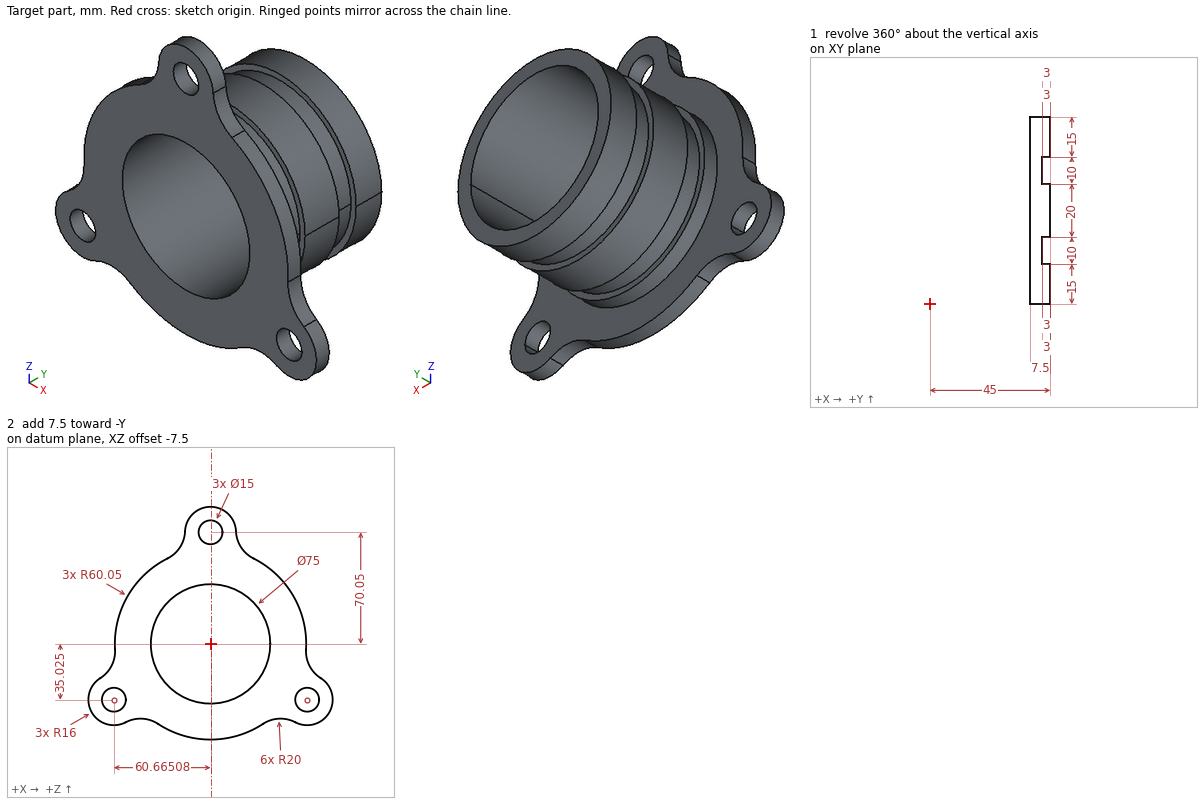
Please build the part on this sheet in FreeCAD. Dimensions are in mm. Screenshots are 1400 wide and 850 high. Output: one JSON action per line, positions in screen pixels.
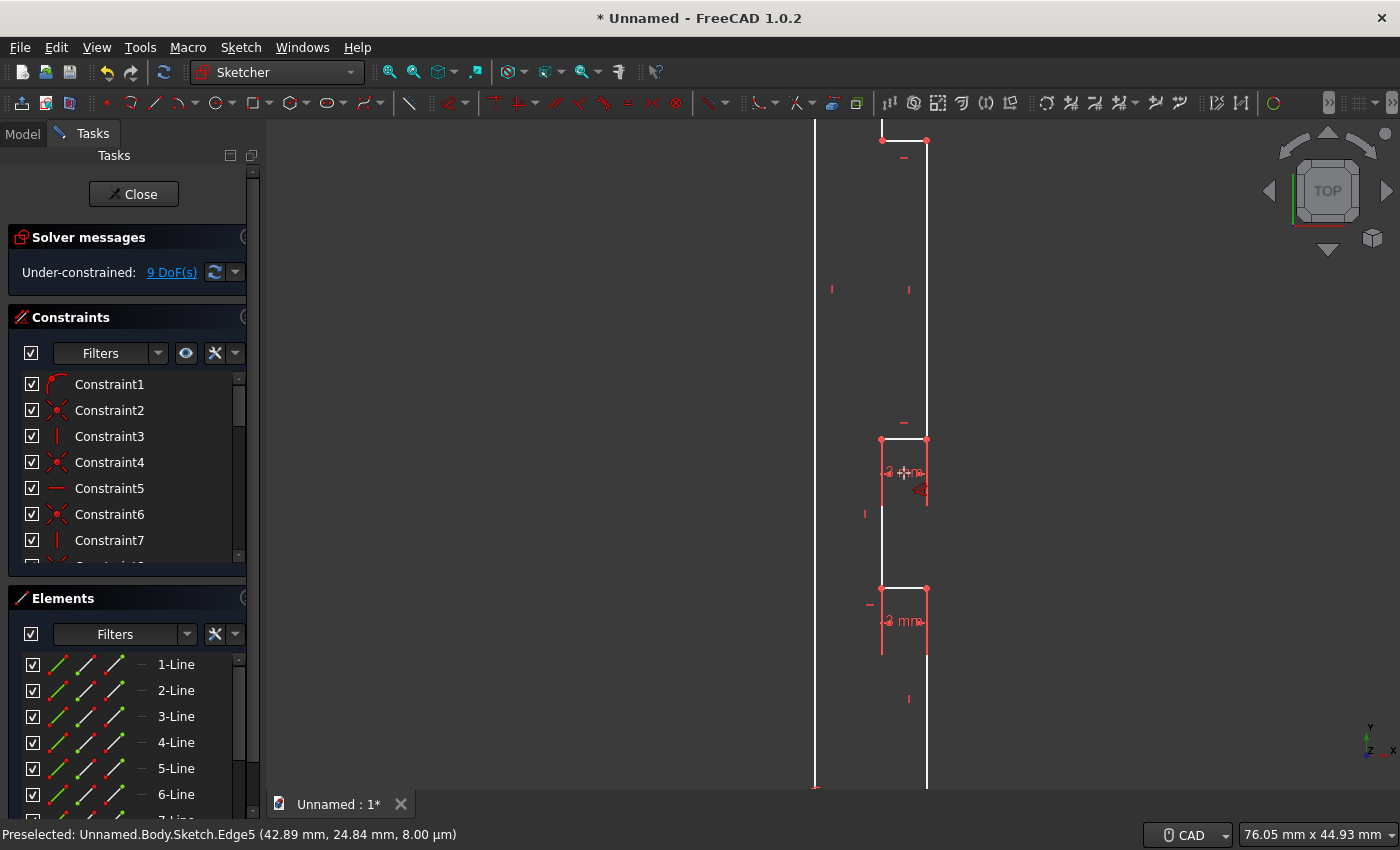
{"action": "scroll", "coordinate": [906, 590], "scroll_direction": "down", "scroll_amount": 4}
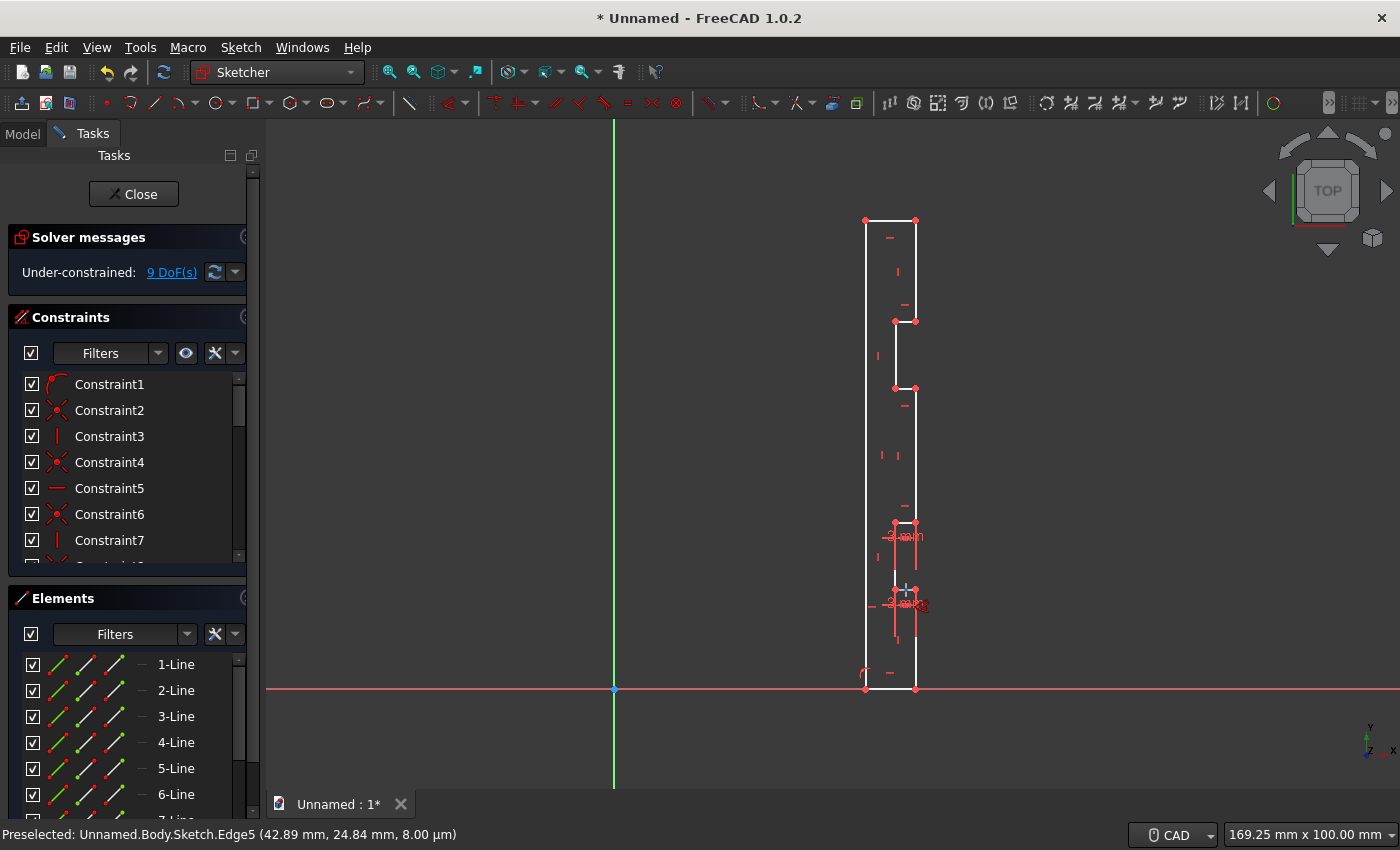
{"action": "scroll", "coordinate": [910, 389], "scroll_direction": "up", "scroll_amount": 5}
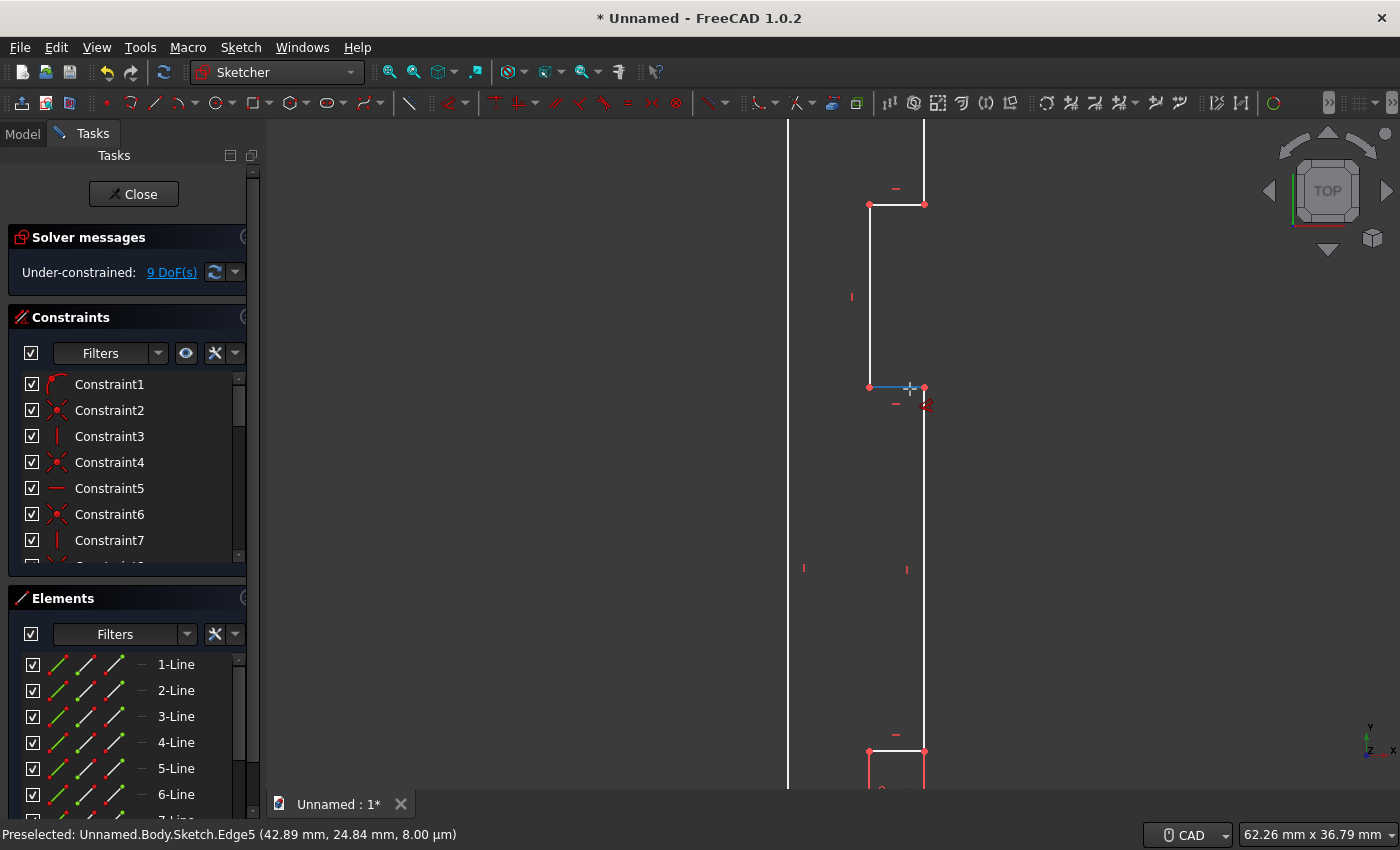
{"action": "left_click", "coordinate": [908, 387]}
{"action": "left_click", "coordinate": [897, 353]}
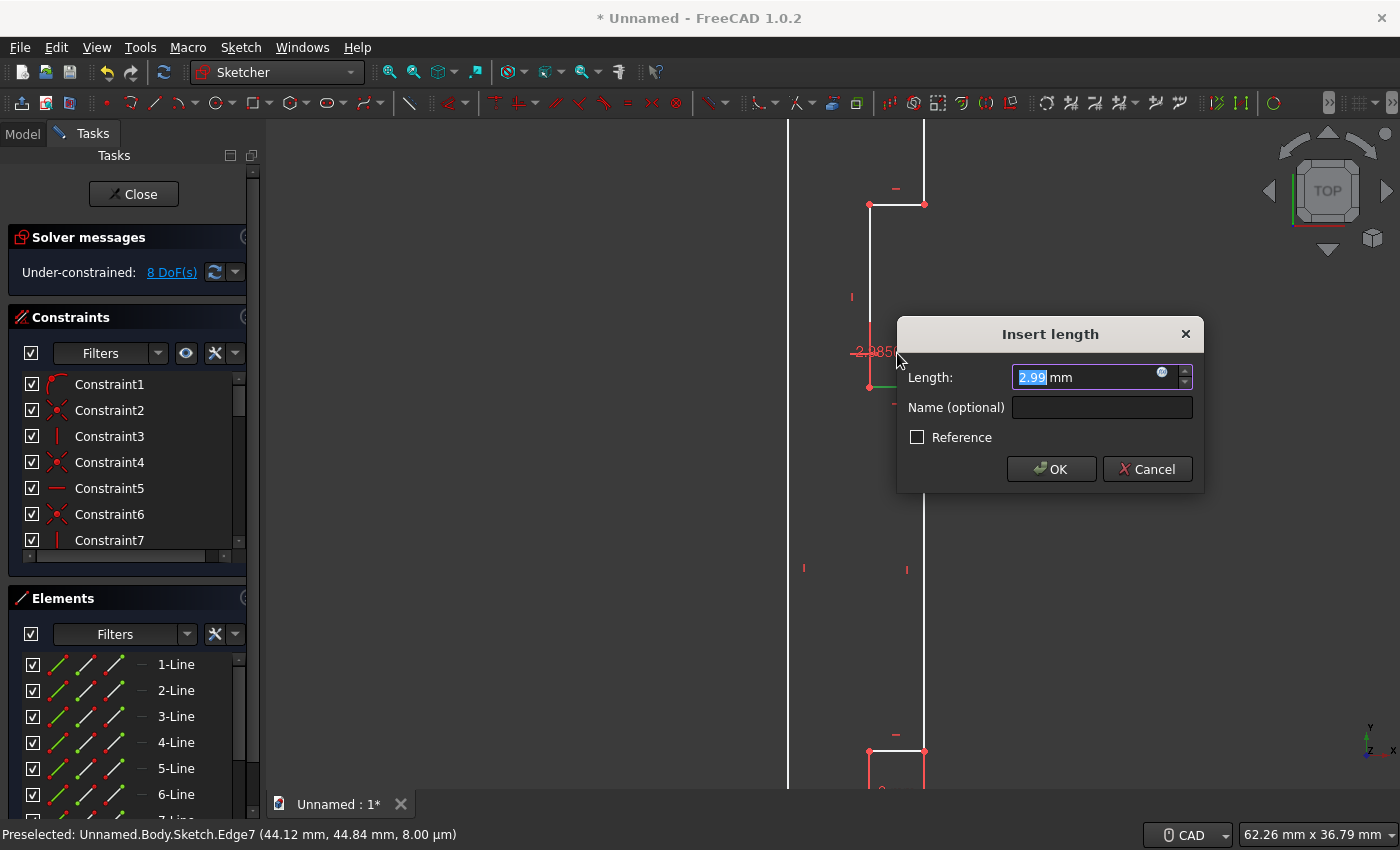
{"action": "type", "text": "3"}
{"action": "key", "text": "Return"}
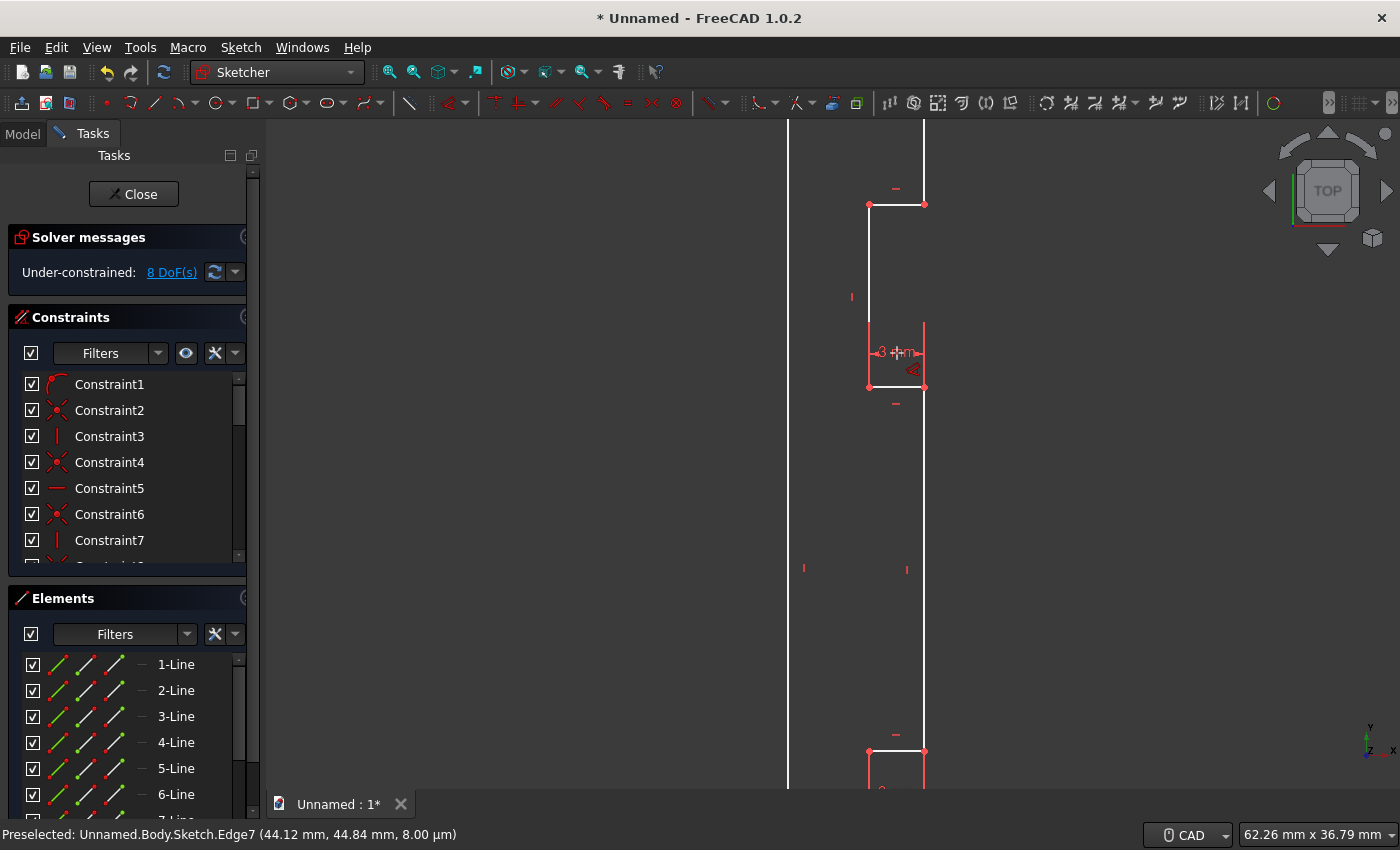
{"action": "left_click", "coordinate": [886, 205]}
{"action": "left_click", "coordinate": [897, 171]}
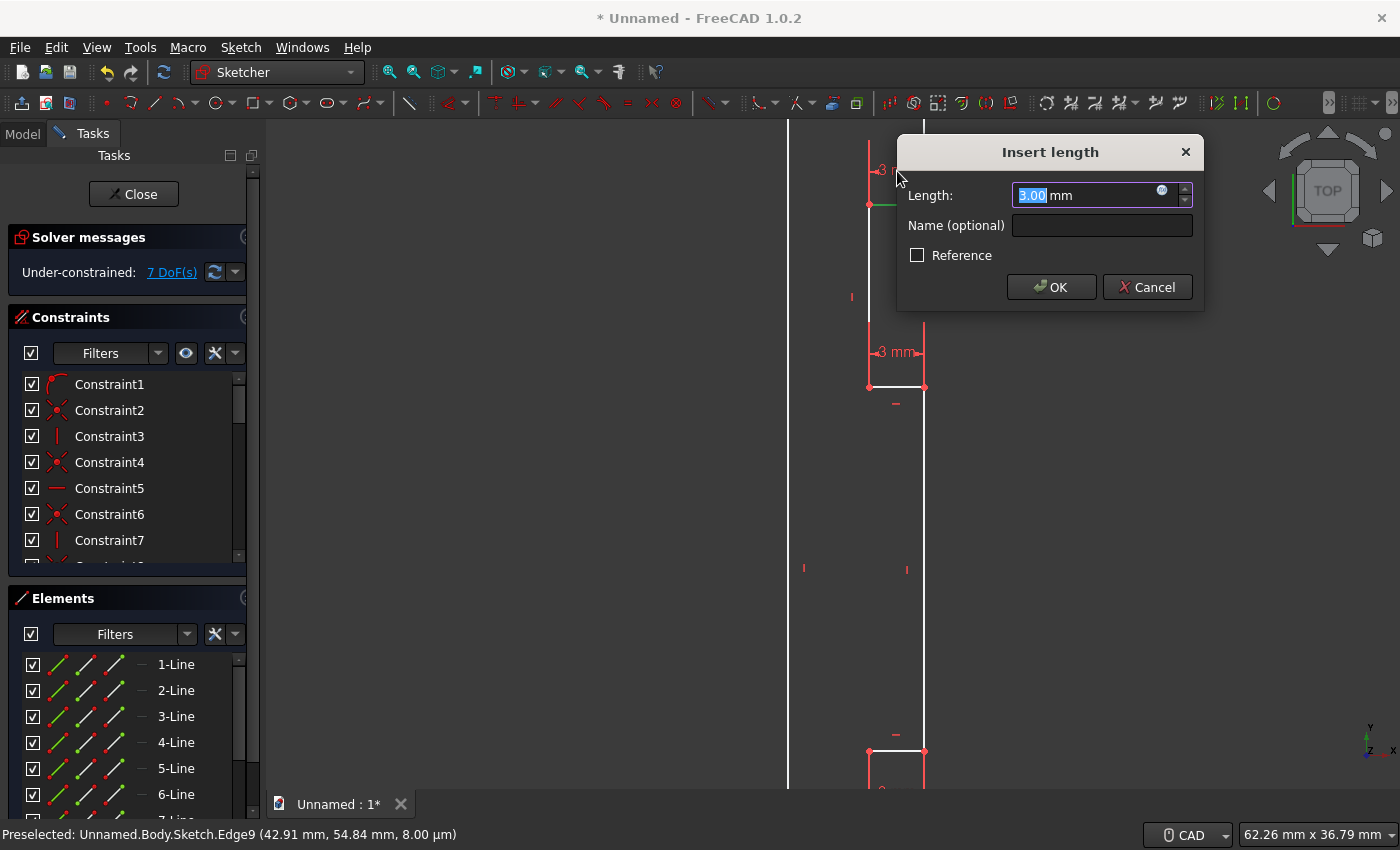
{"action": "type", "text": "3"}
{"action": "key", "text": "Return"}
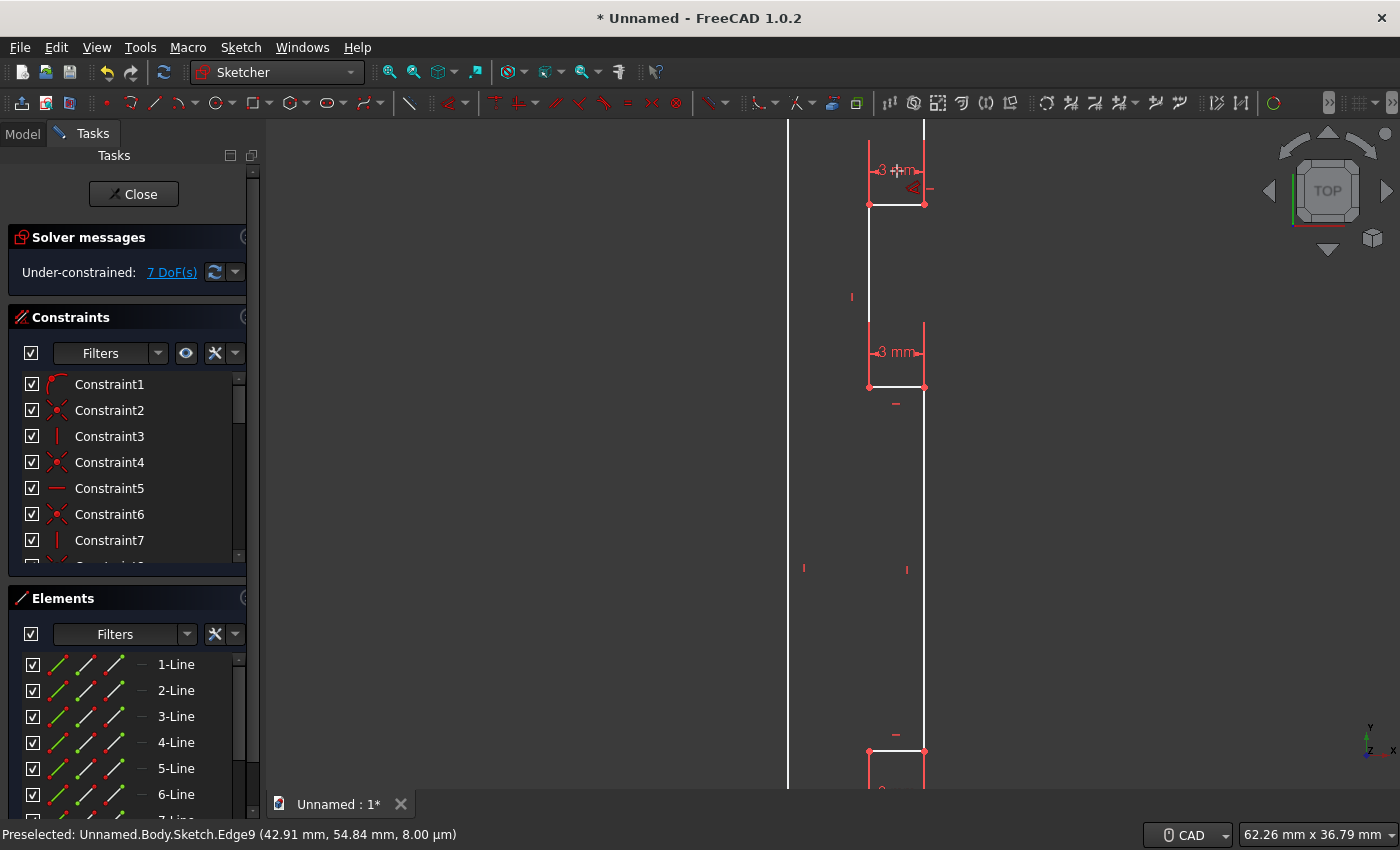
{"action": "scroll", "coordinate": [910, 389], "scroll_direction": "down", "scroll_amount": 5}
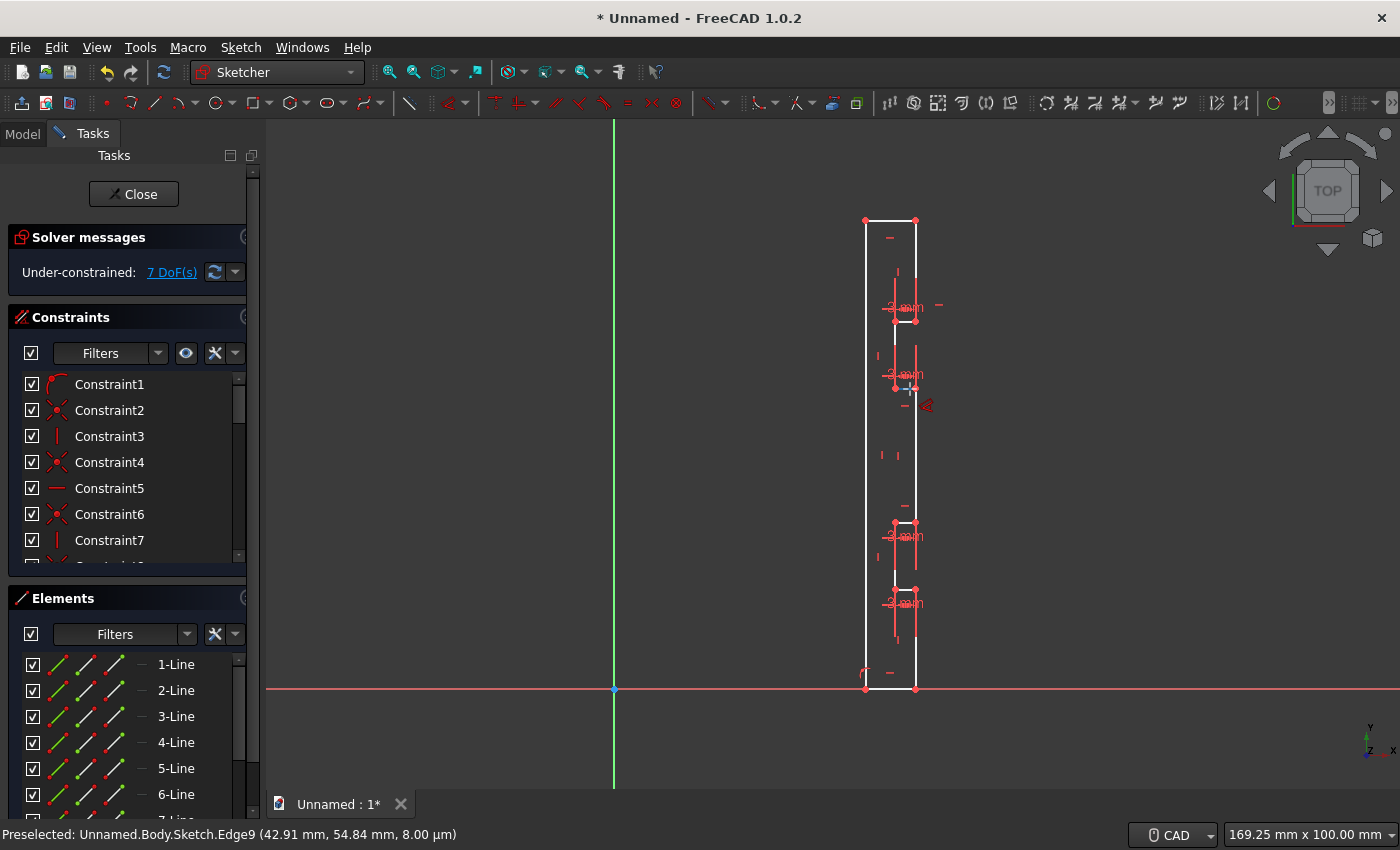
{"action": "left_click", "coordinate": [916, 659]}
{"action": "left_click", "coordinate": [950, 639]}